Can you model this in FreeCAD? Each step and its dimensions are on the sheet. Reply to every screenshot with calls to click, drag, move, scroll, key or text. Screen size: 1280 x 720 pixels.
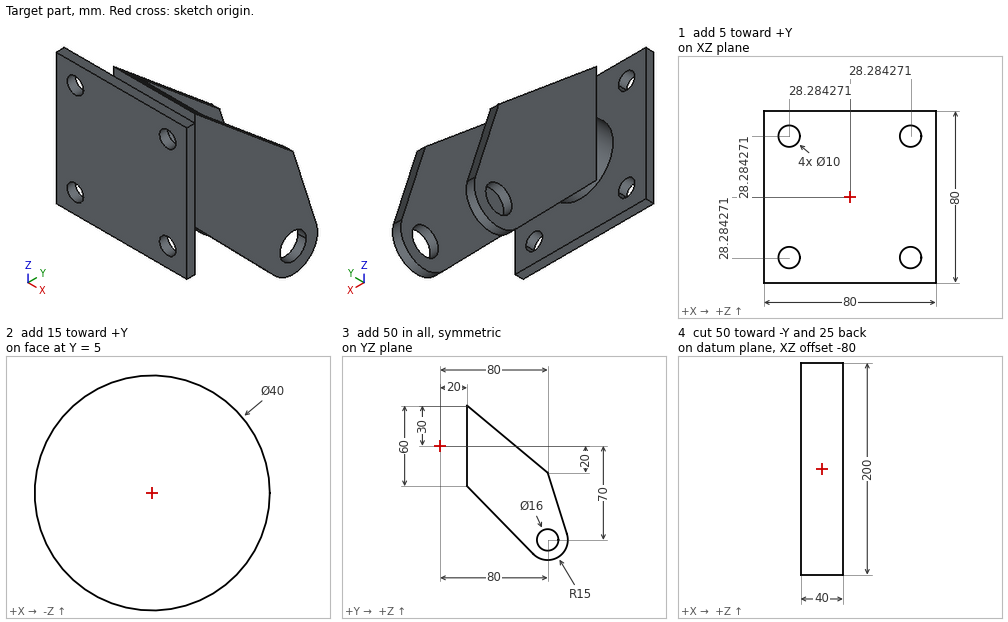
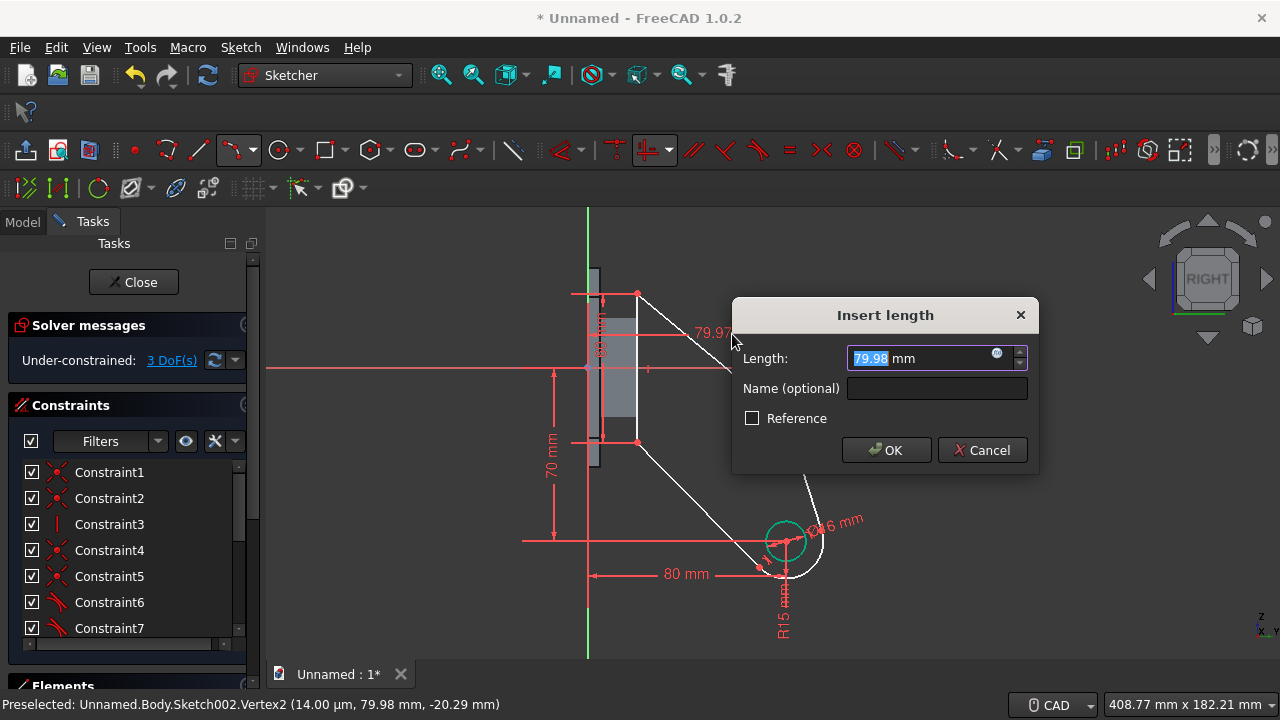
text(80)
key(Return)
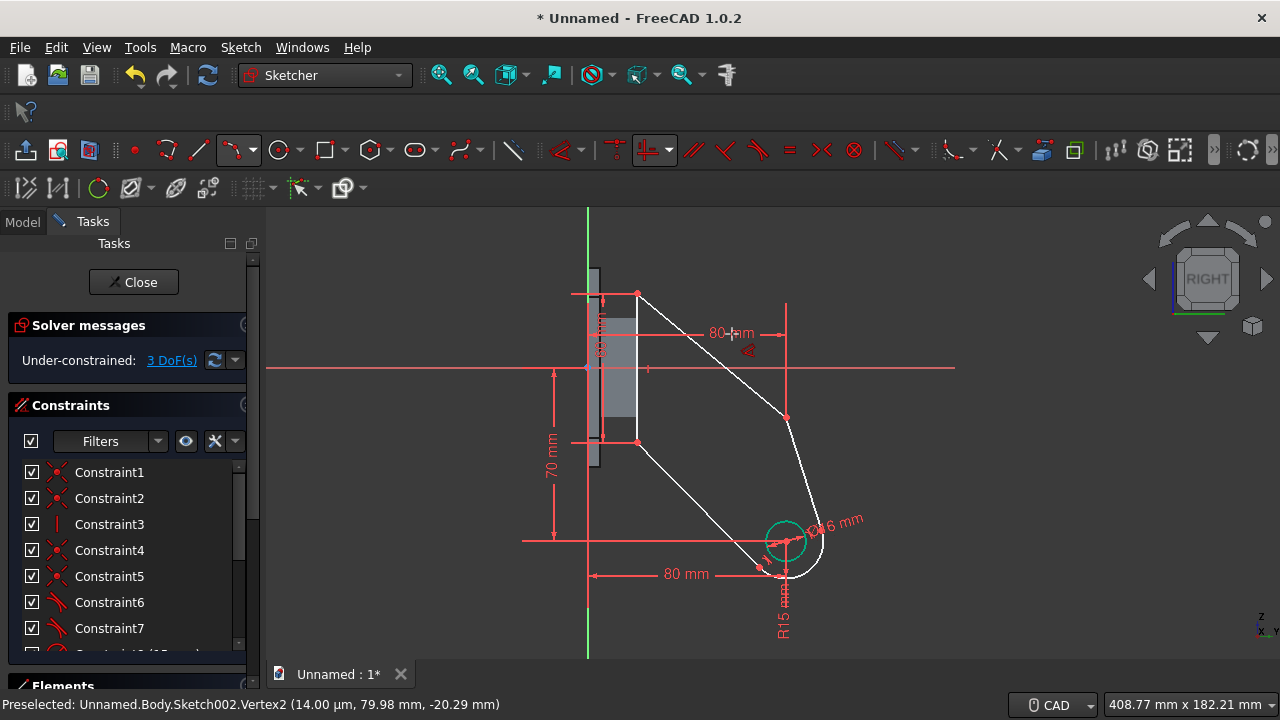
click(786, 418)
click(554, 393)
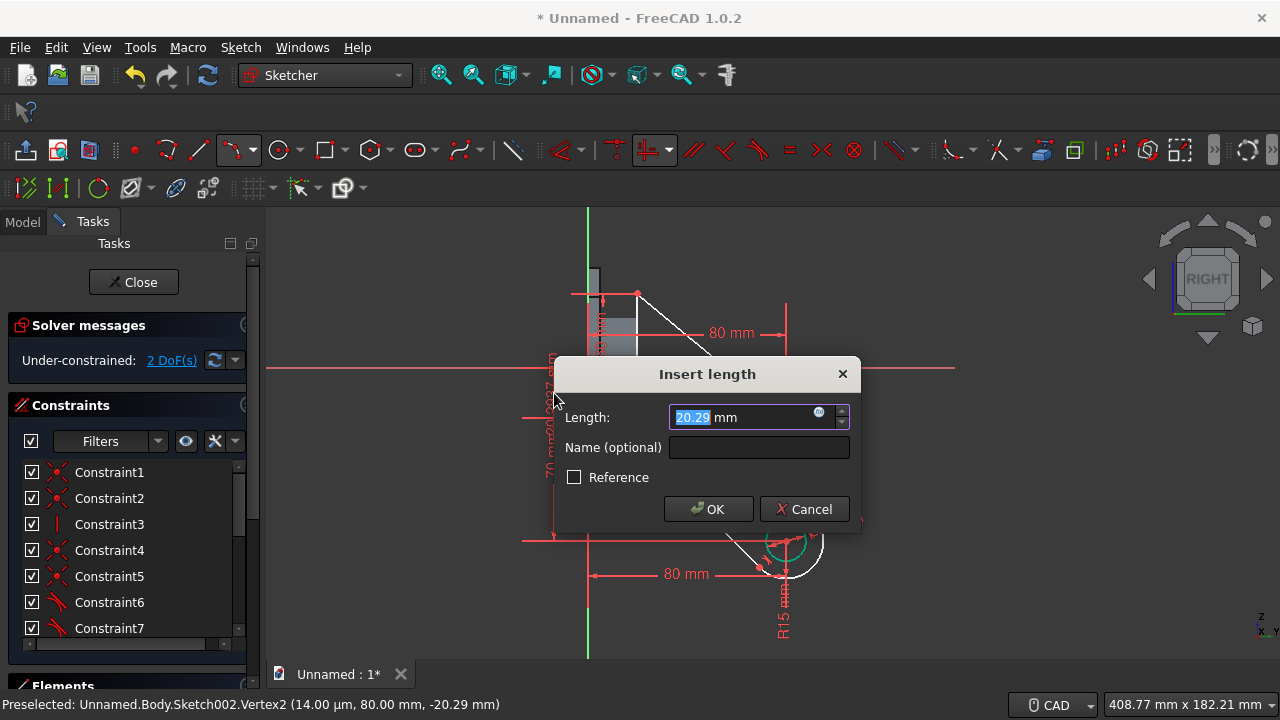
text(20)
key(Return)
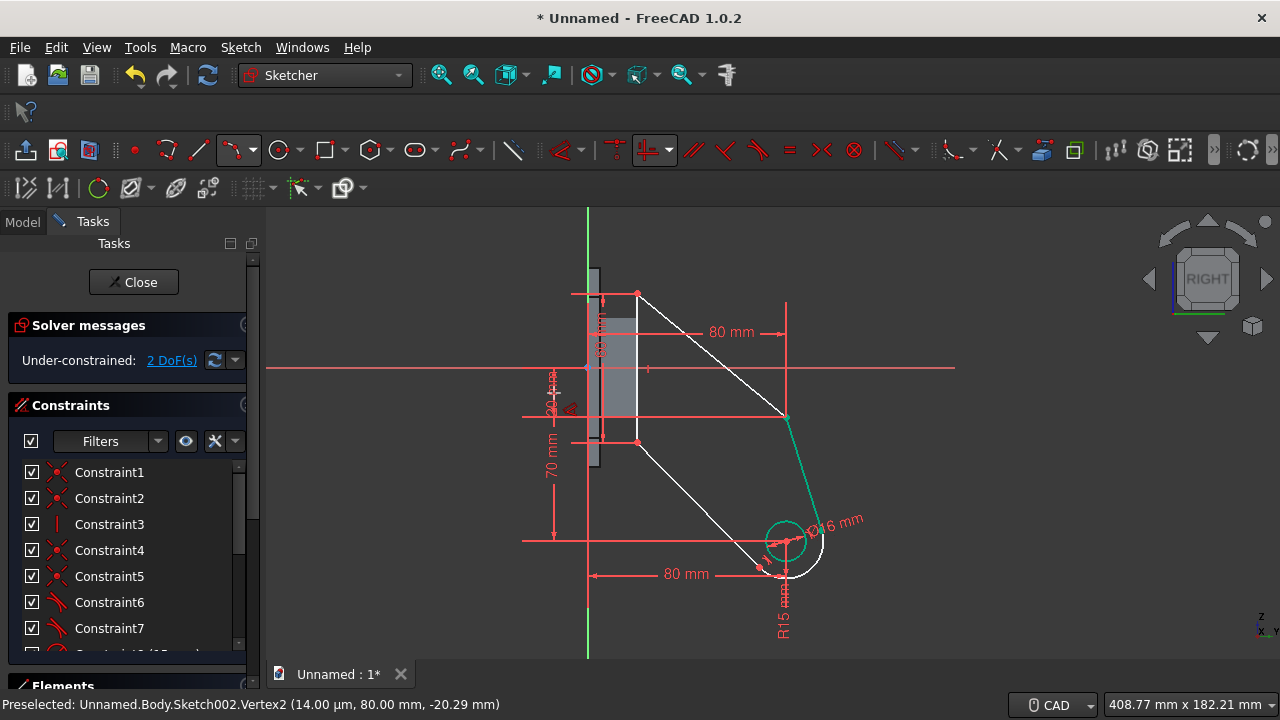
click(637, 294)
click(612, 260)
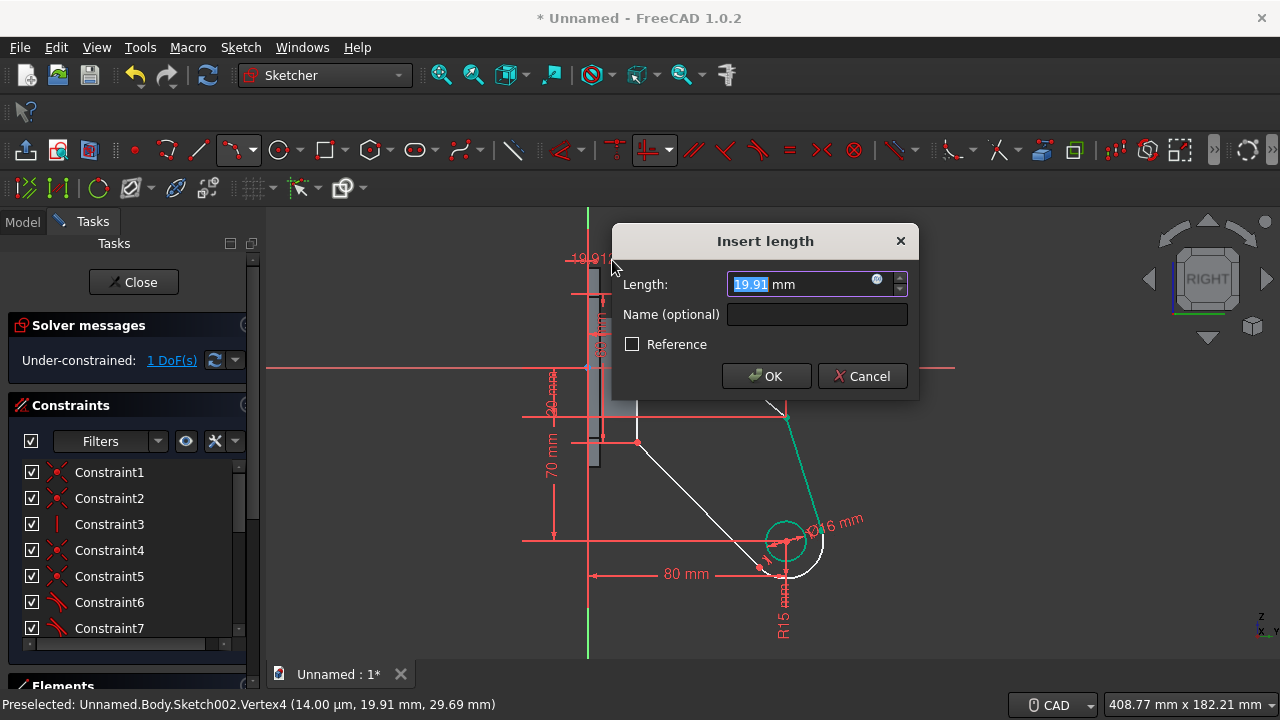
text(20)
key(Return)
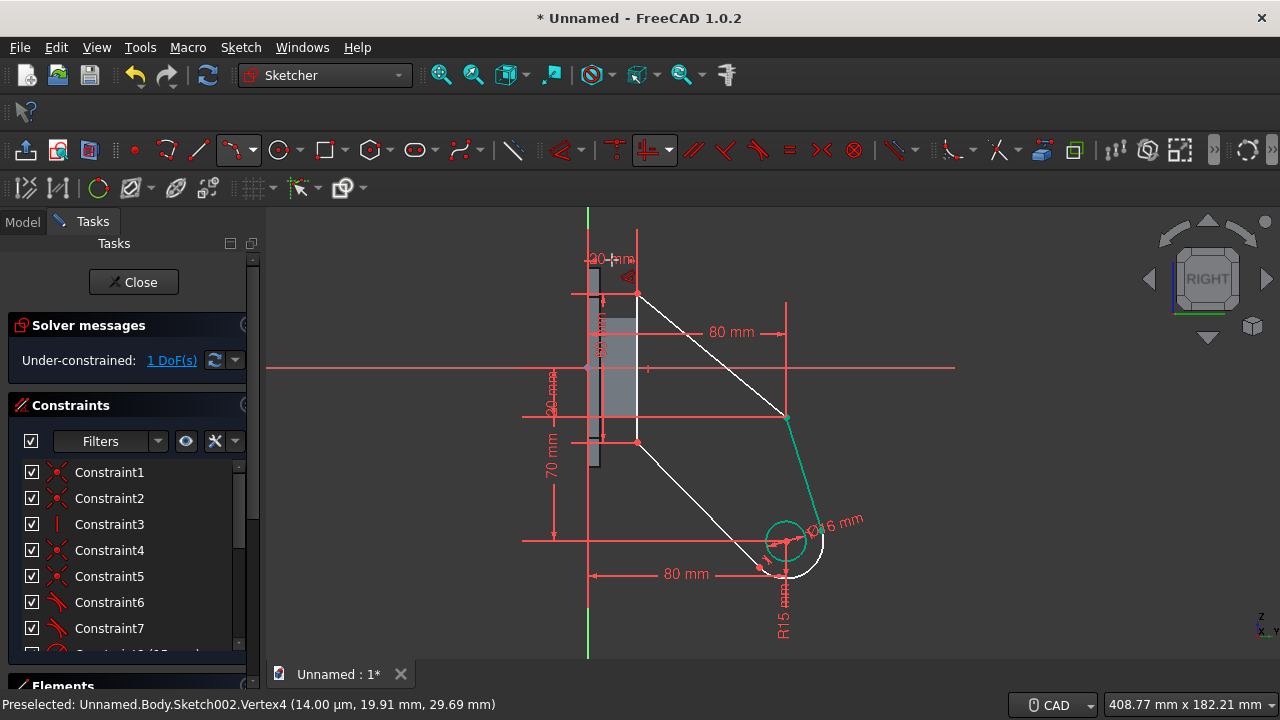
click(637, 294)
click(554, 314)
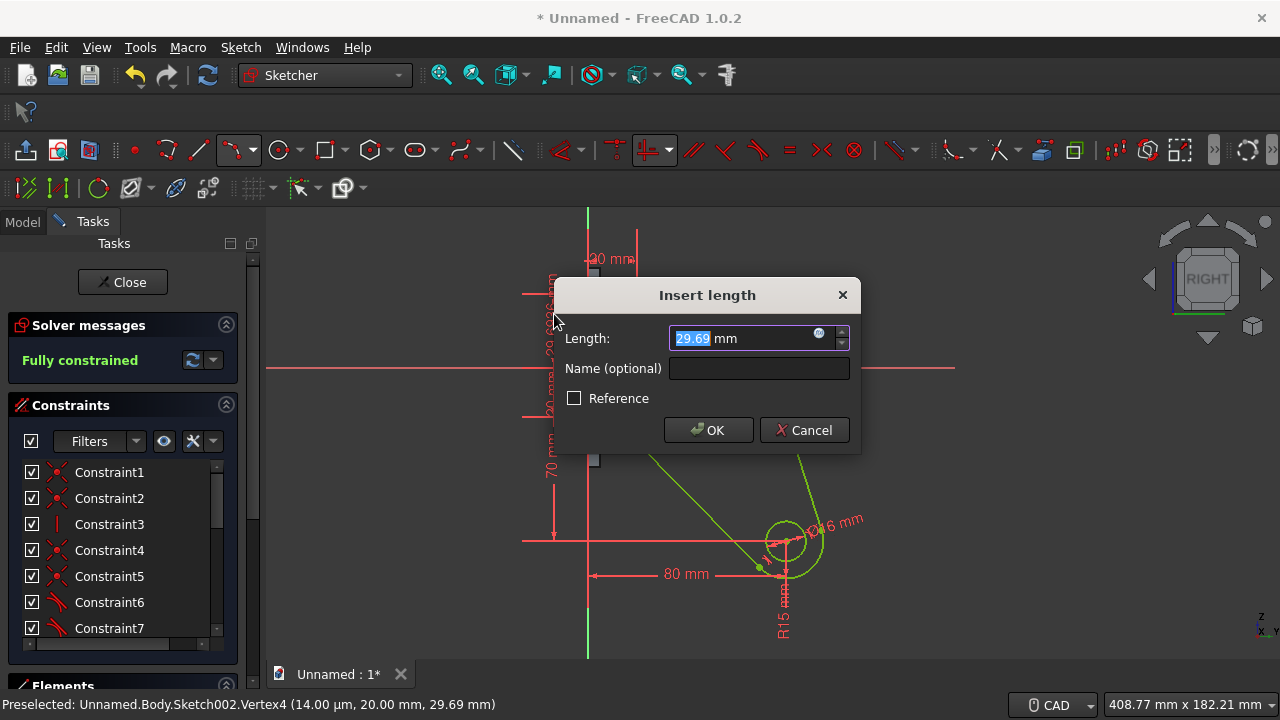
text(30)
key(Return)
key(Escape)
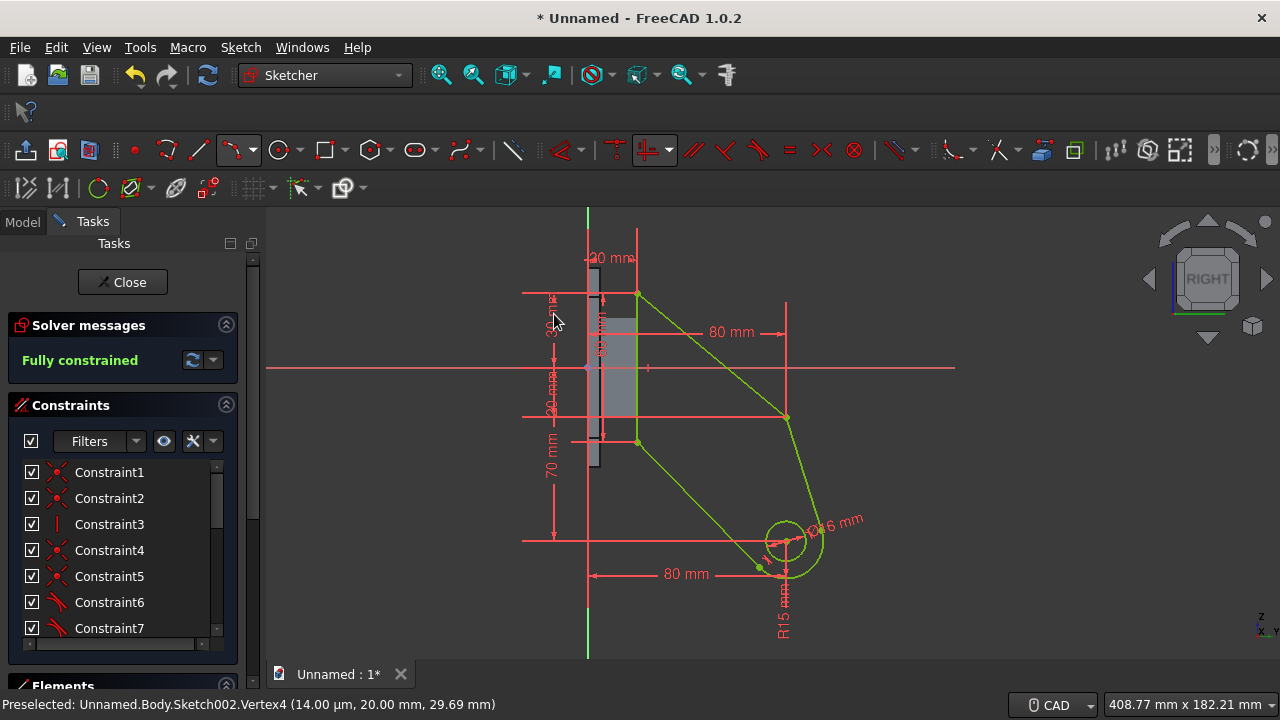
click(123, 282)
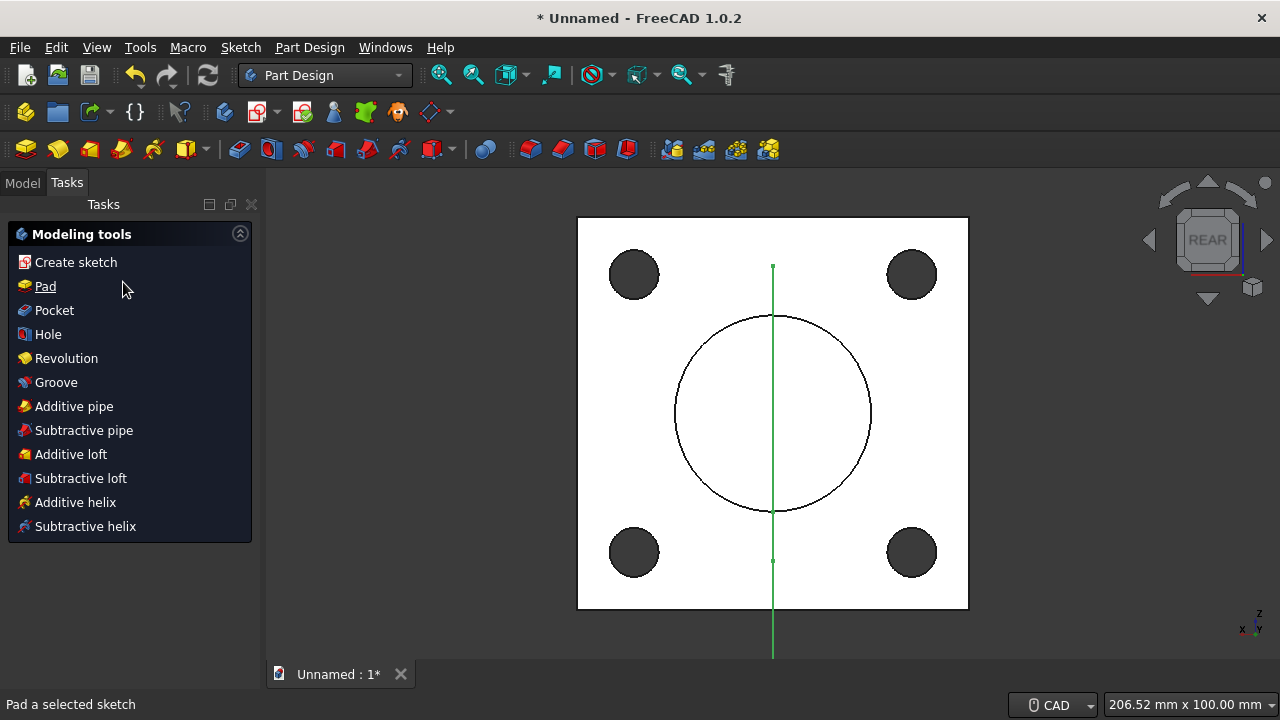
click(26, 150)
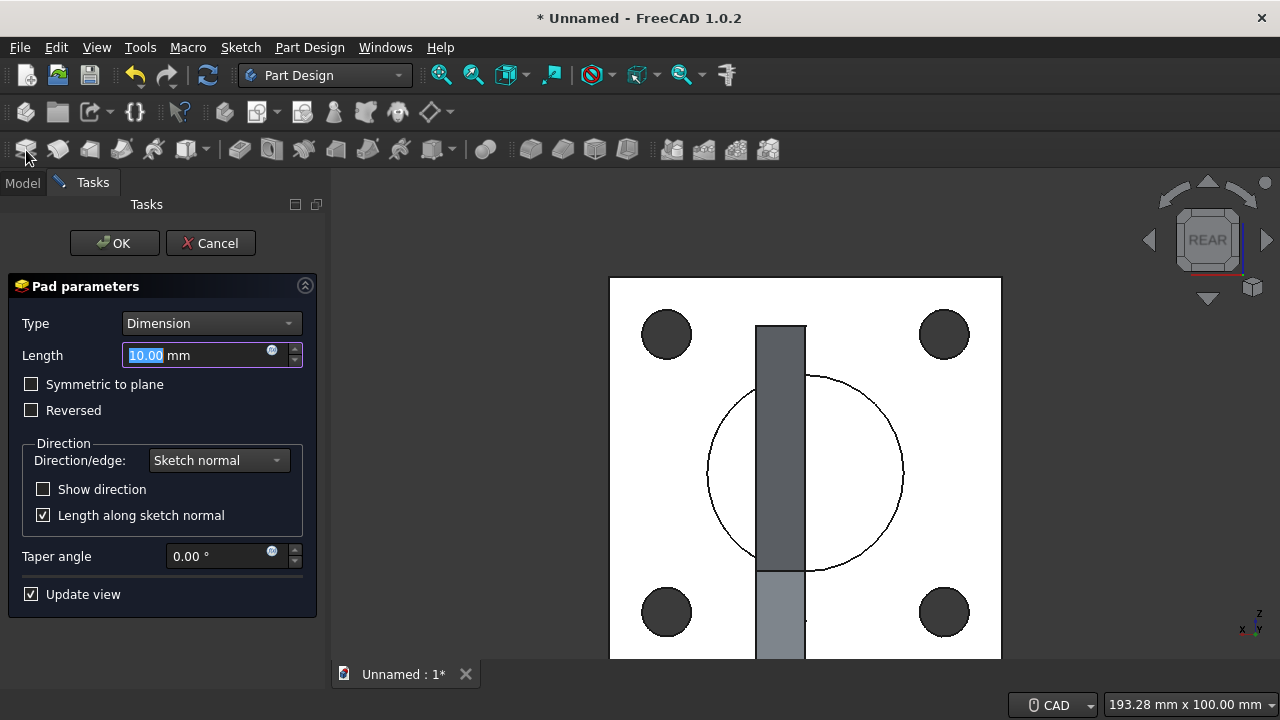
text(50)
key(Tab)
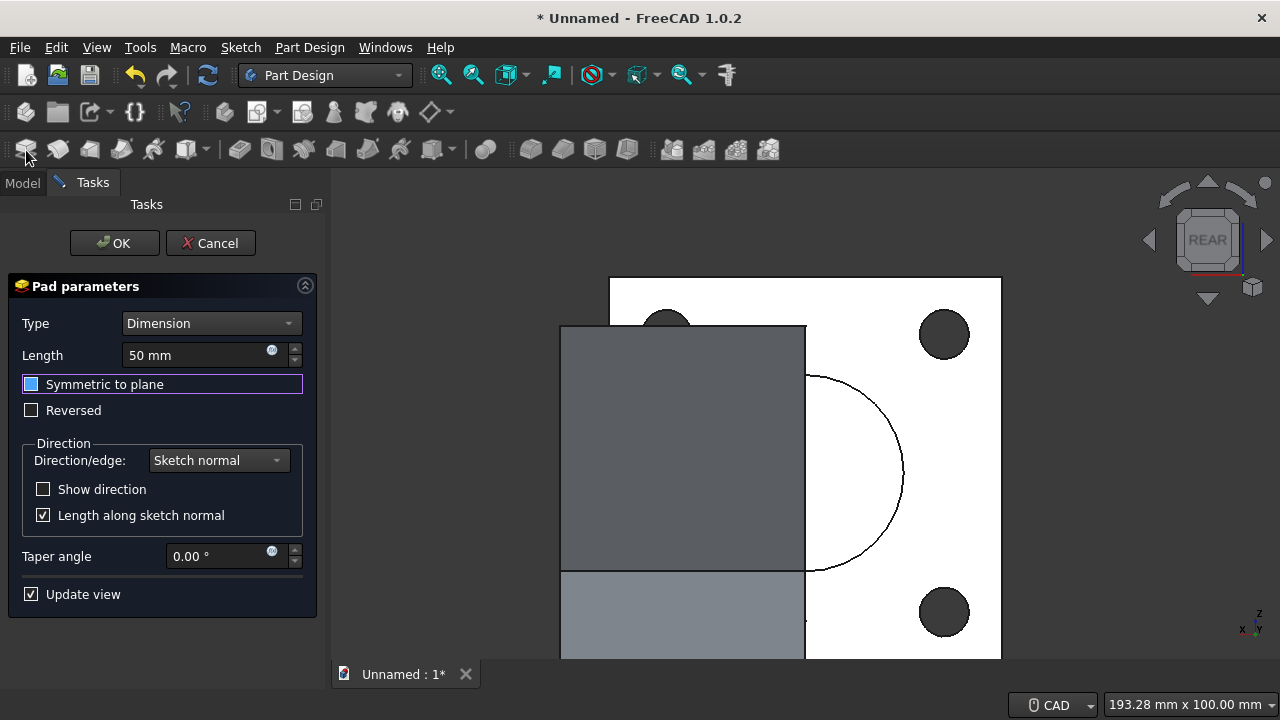
click(30, 384)